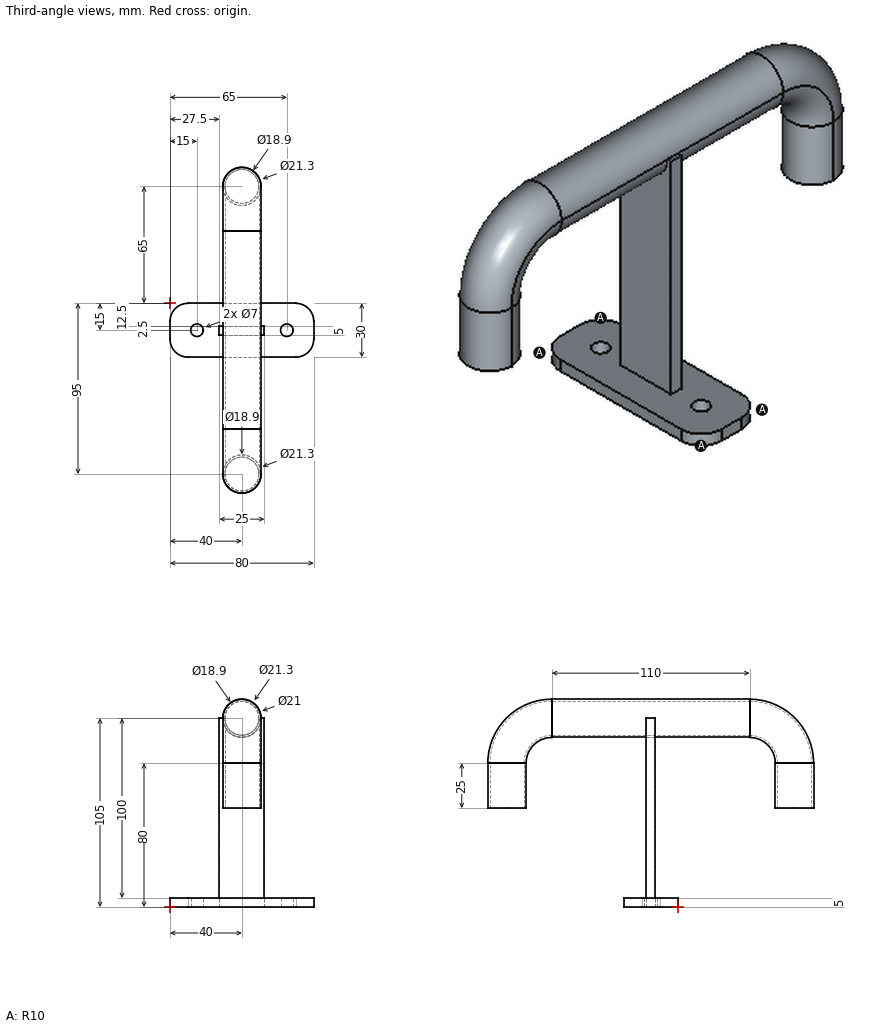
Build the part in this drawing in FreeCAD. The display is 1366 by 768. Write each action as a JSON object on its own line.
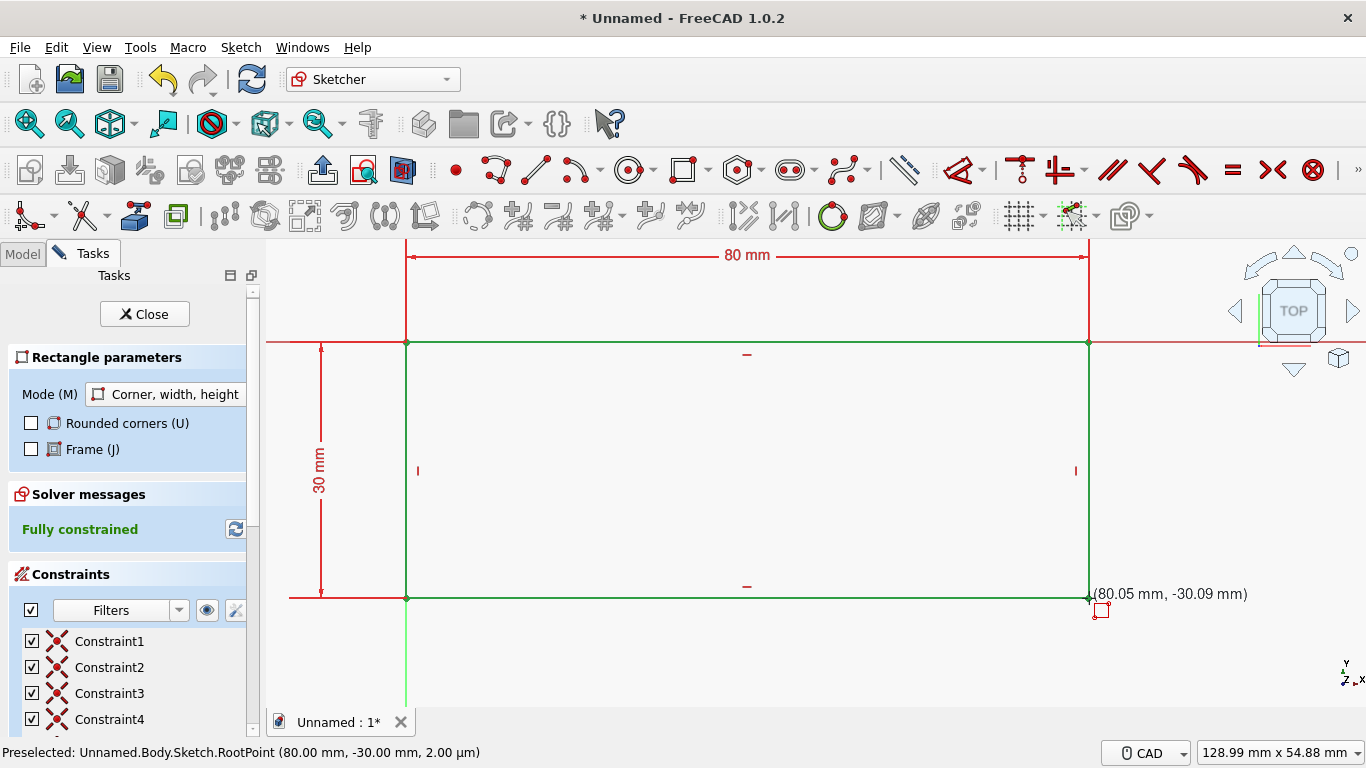
{"action": "left_click", "coordinate": [641, 449]}
{"action": "mouse_move", "coordinate": [854, 492]}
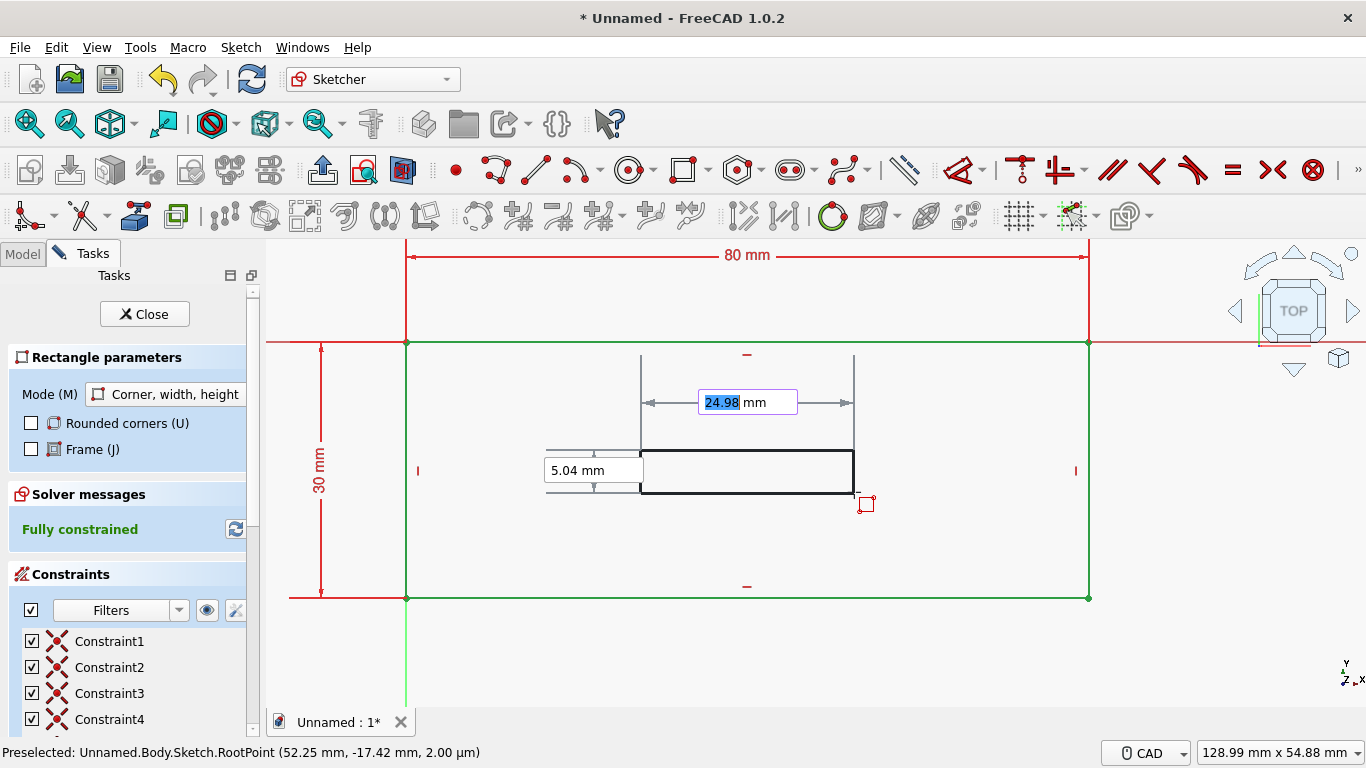
{"action": "type", "text": "25"}
{"action": "key", "text": "Tab"}
{"action": "type", "text": "5"}
{"action": "key", "text": "Return"}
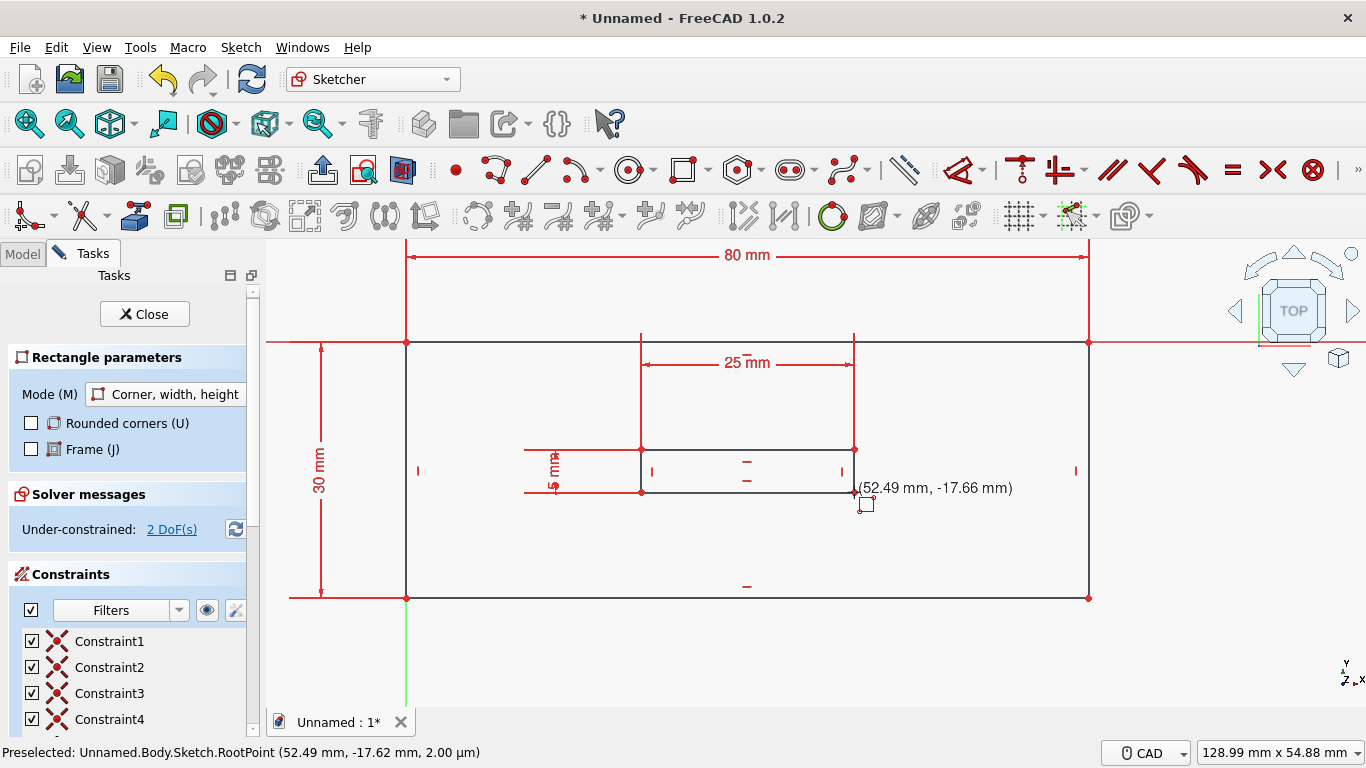
{"action": "left_click", "coordinate": [630, 170]}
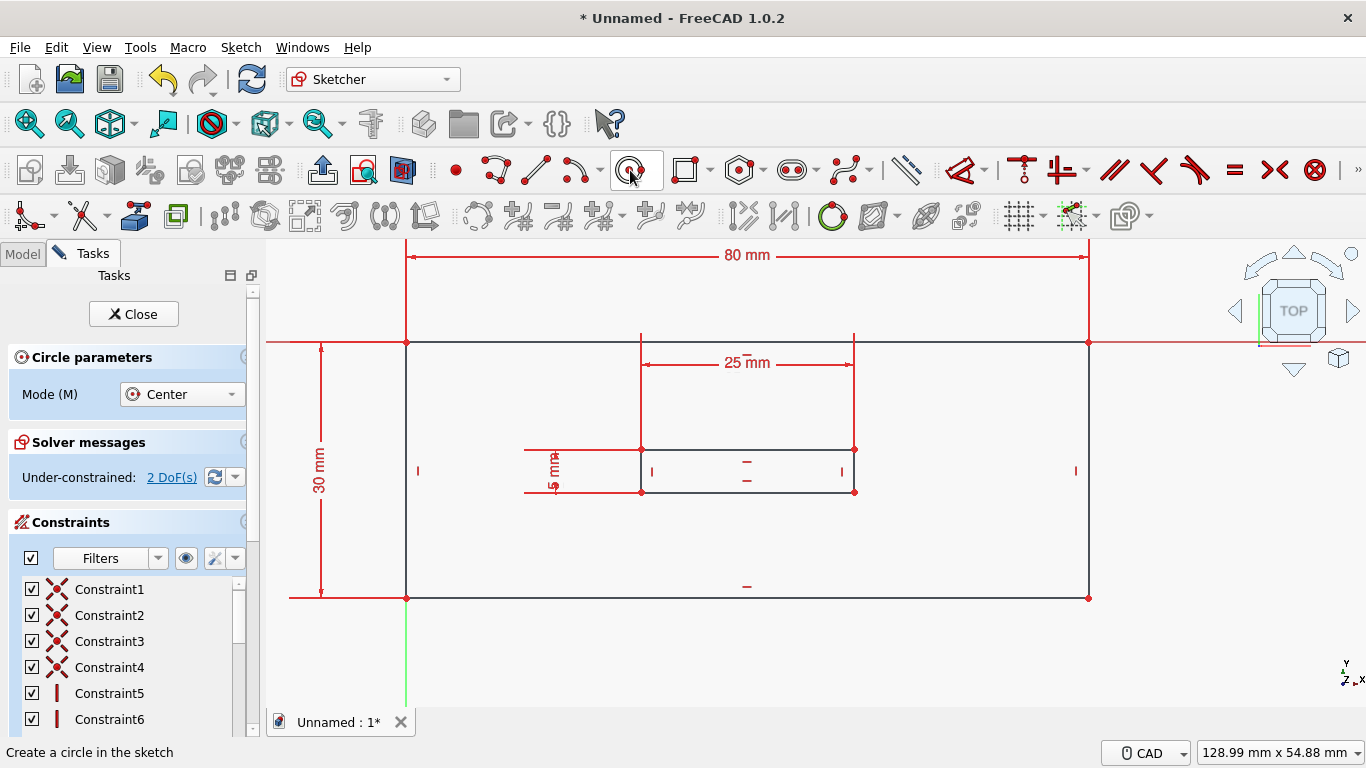
{"action": "left_click", "coordinate": [534, 470]}
{"action": "mouse_move", "coordinate": [555, 449]}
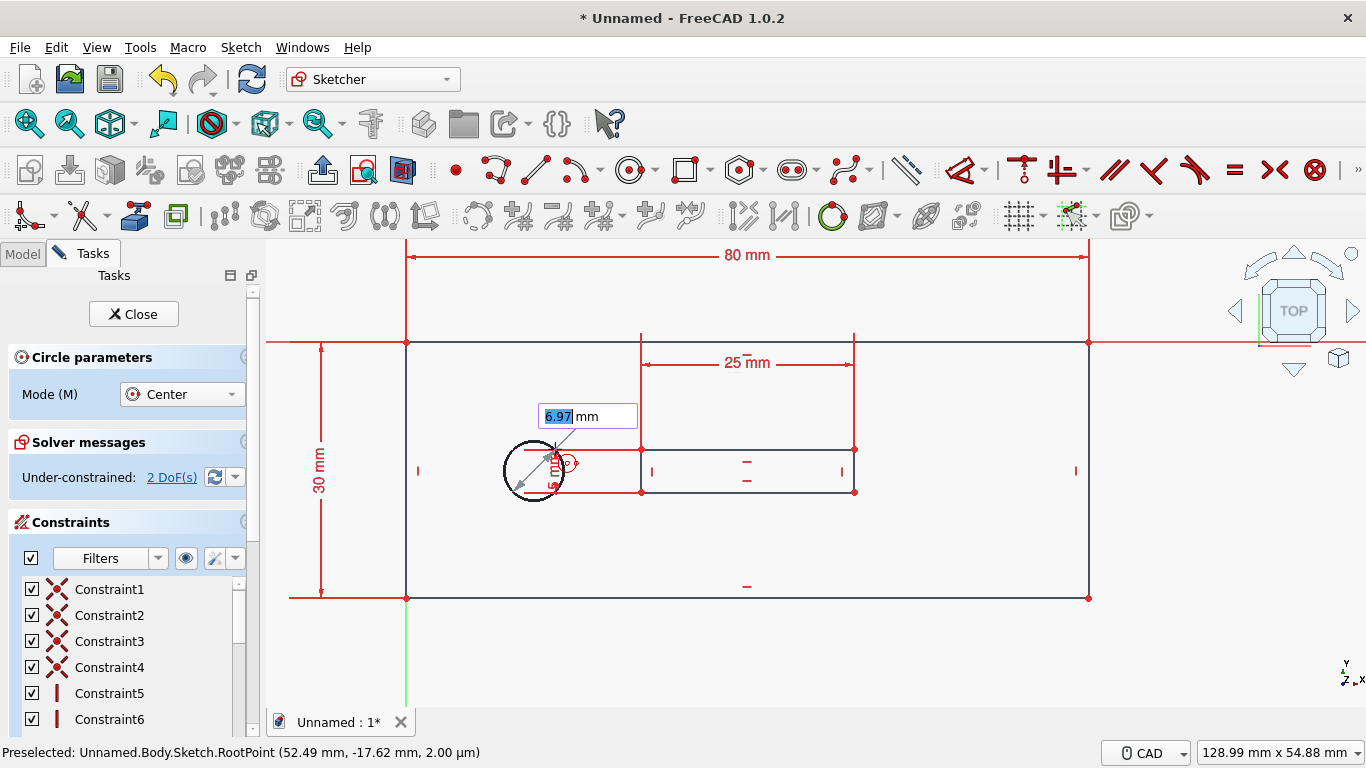
{"action": "type", "text": "7"}
{"action": "key", "text": "Return"}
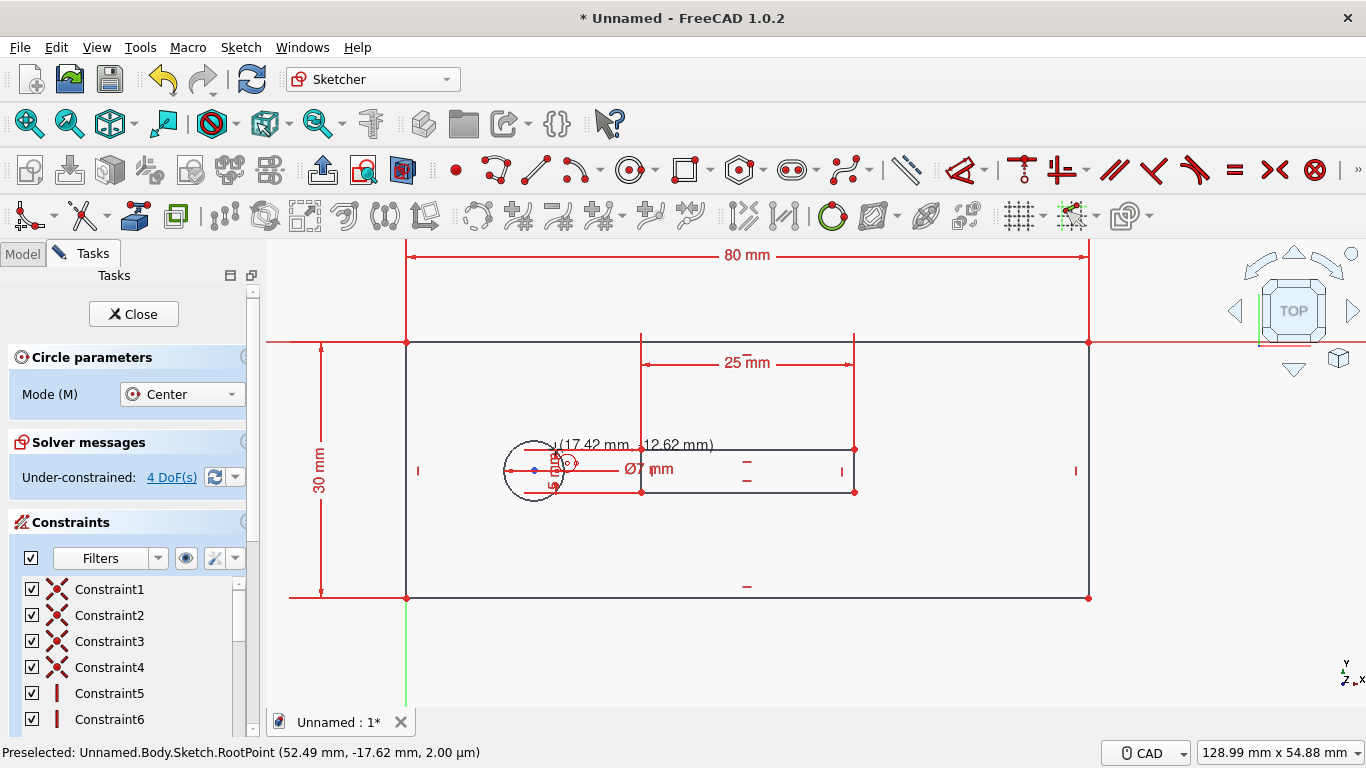
{"action": "left_click", "coordinate": [961, 470]}
{"action": "mouse_move", "coordinate": [982, 449]}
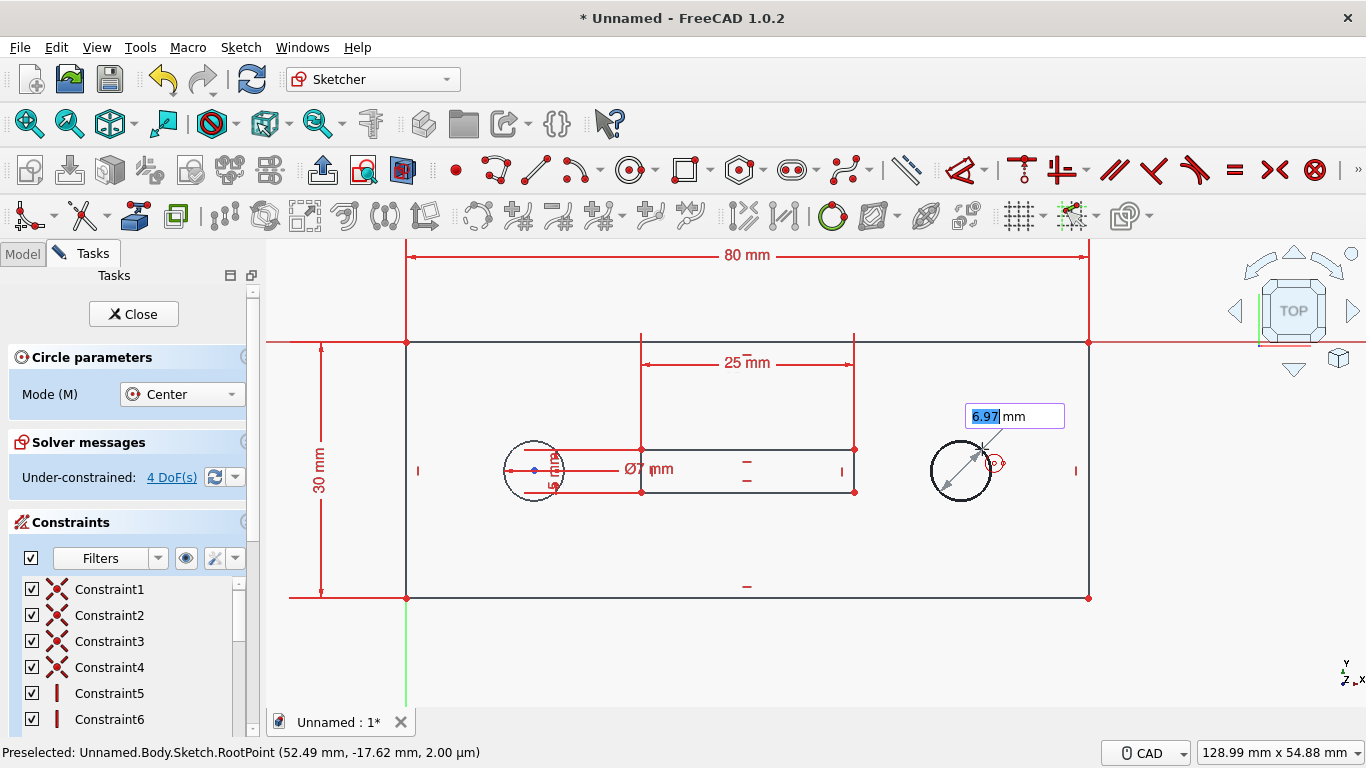
{"action": "type", "text": "7"}
{"action": "key", "text": "Return"}
{"action": "key", "text": "Escape"}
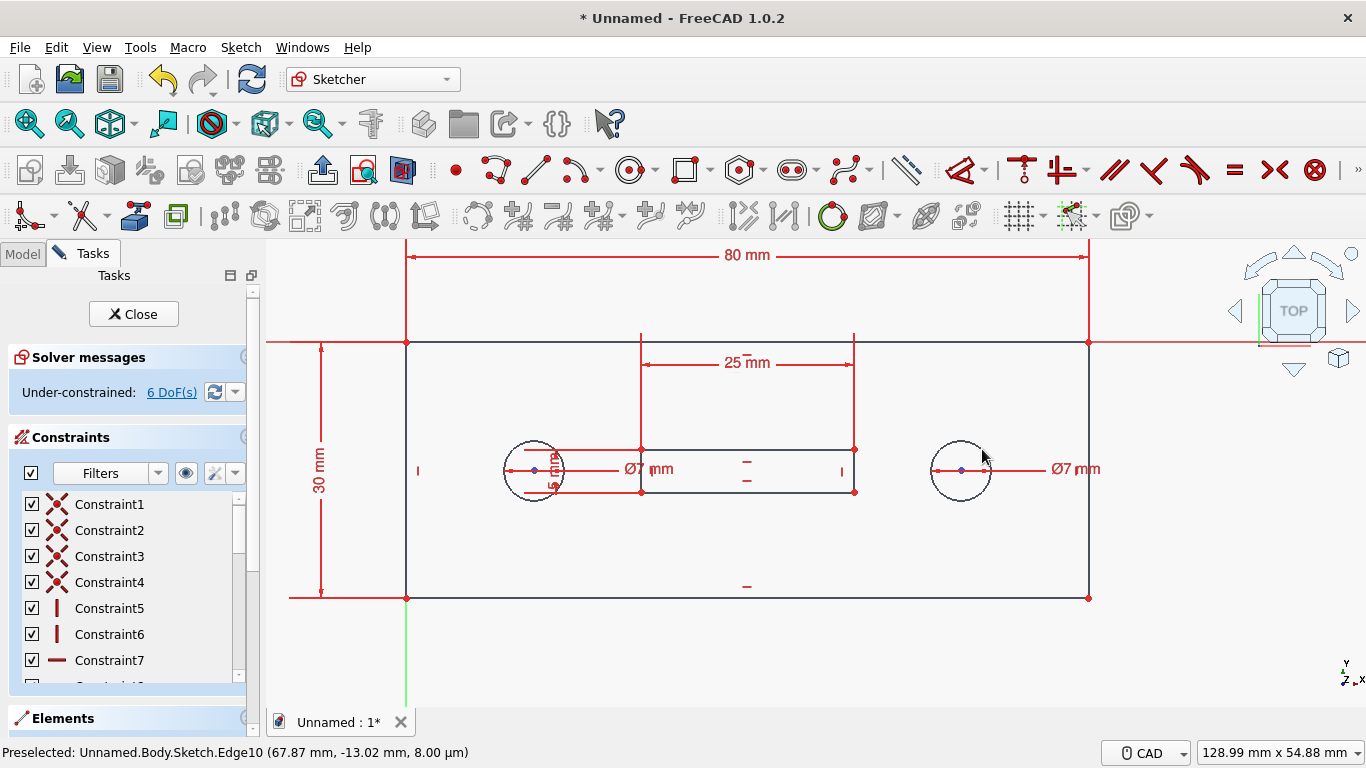
{"action": "left_click", "coordinate": [960, 170]}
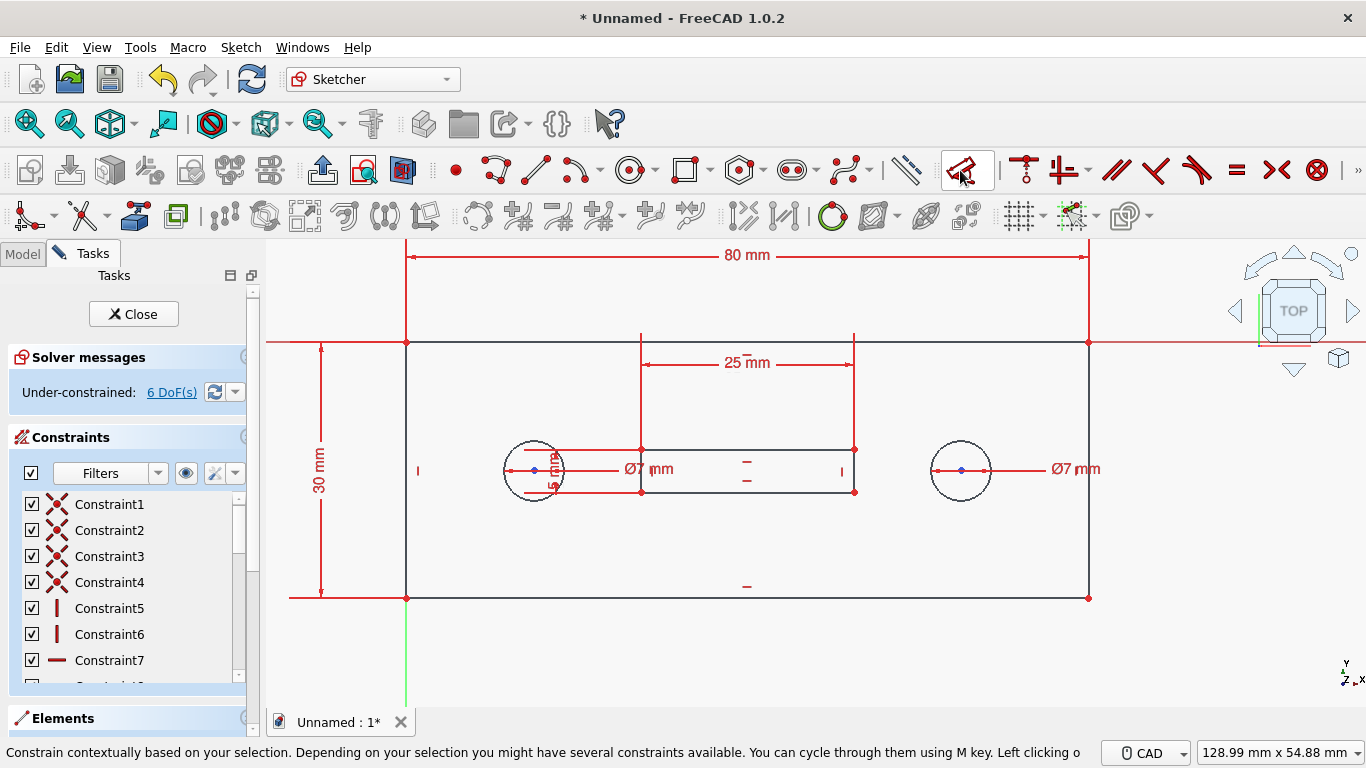
{"action": "left_click", "coordinate": [534, 471]}
{"action": "left_click", "coordinate": [470, 308]}